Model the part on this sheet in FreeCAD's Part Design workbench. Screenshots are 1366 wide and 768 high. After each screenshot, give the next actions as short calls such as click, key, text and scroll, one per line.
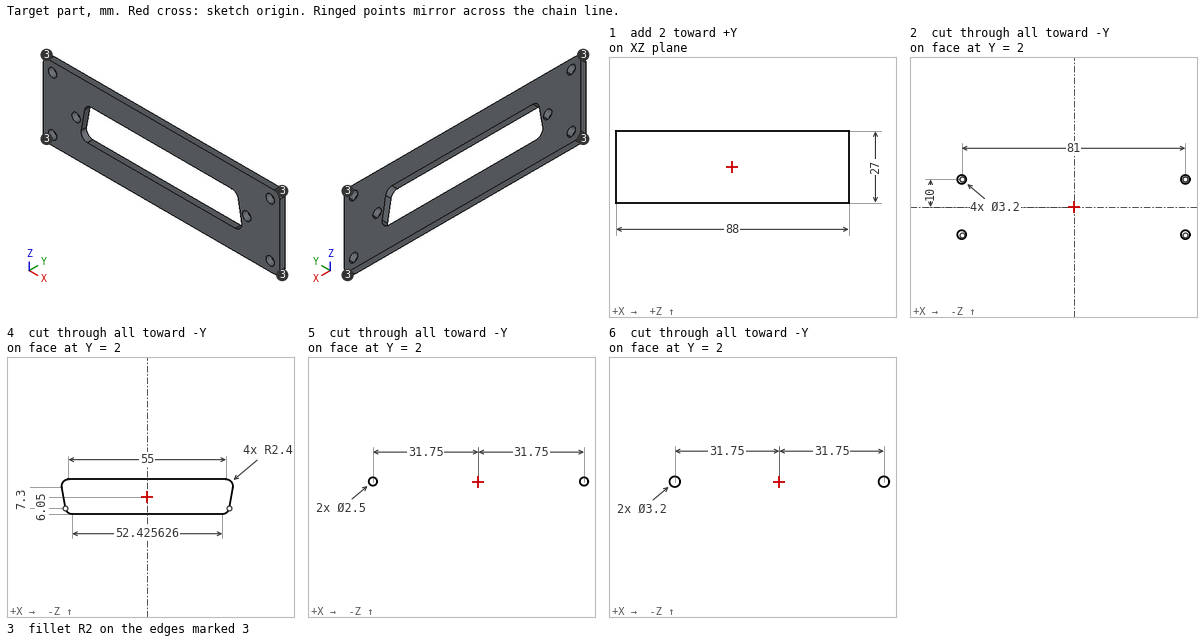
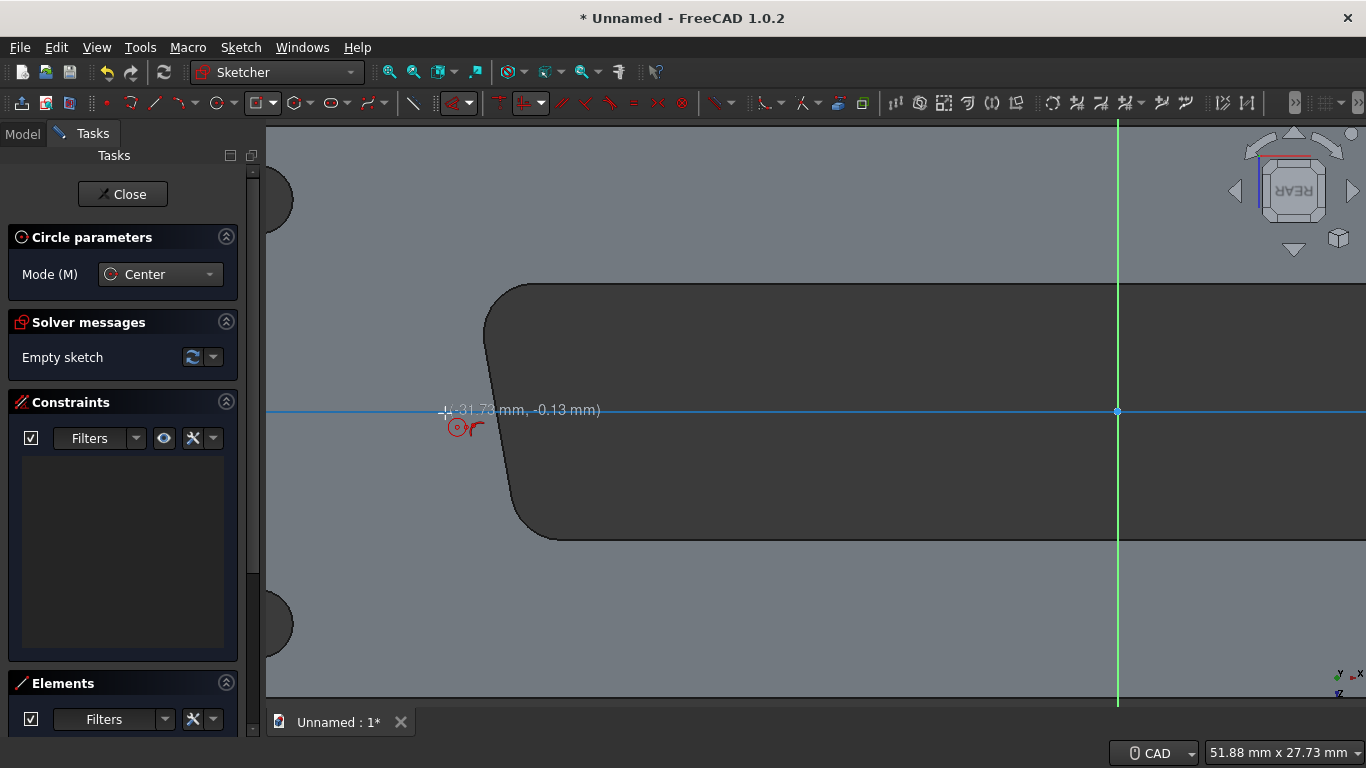
click(444, 412)
click(463, 393)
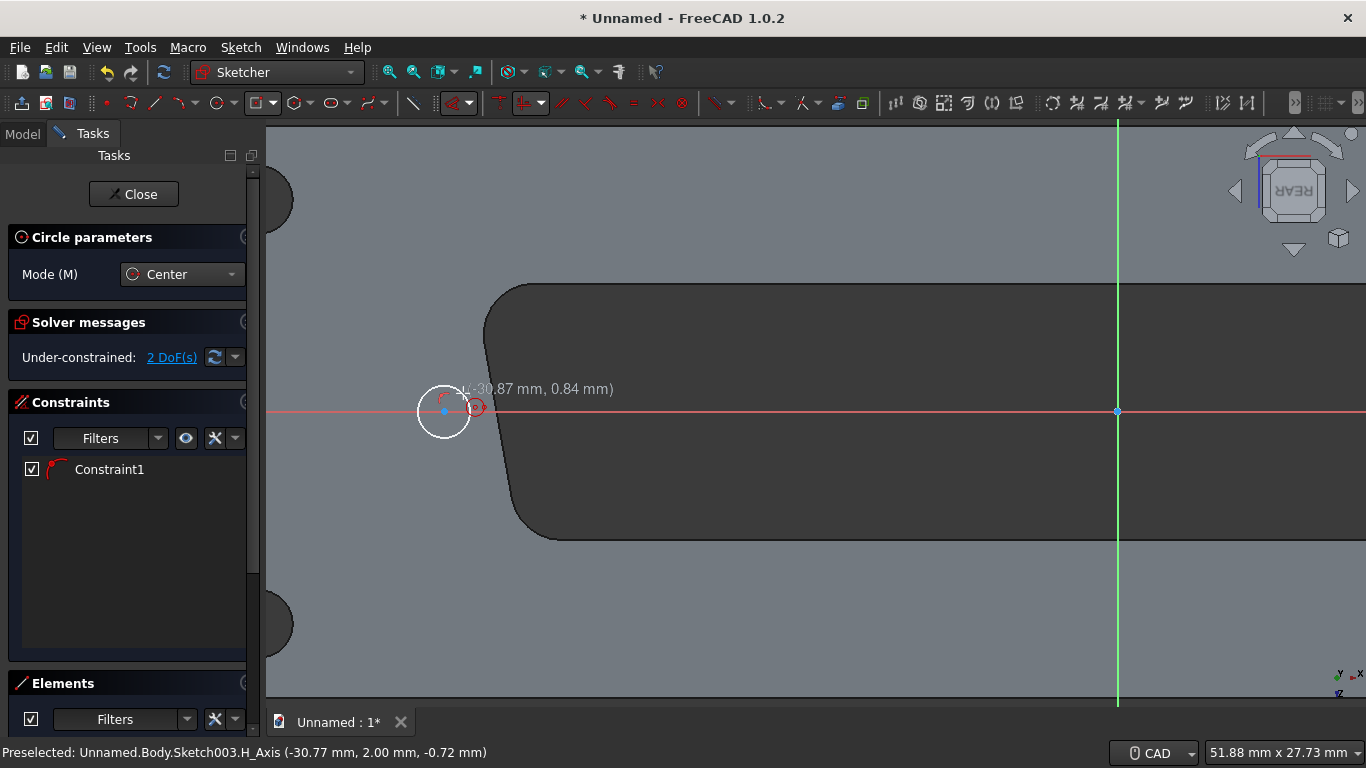
scroll(445, 414, down, 4)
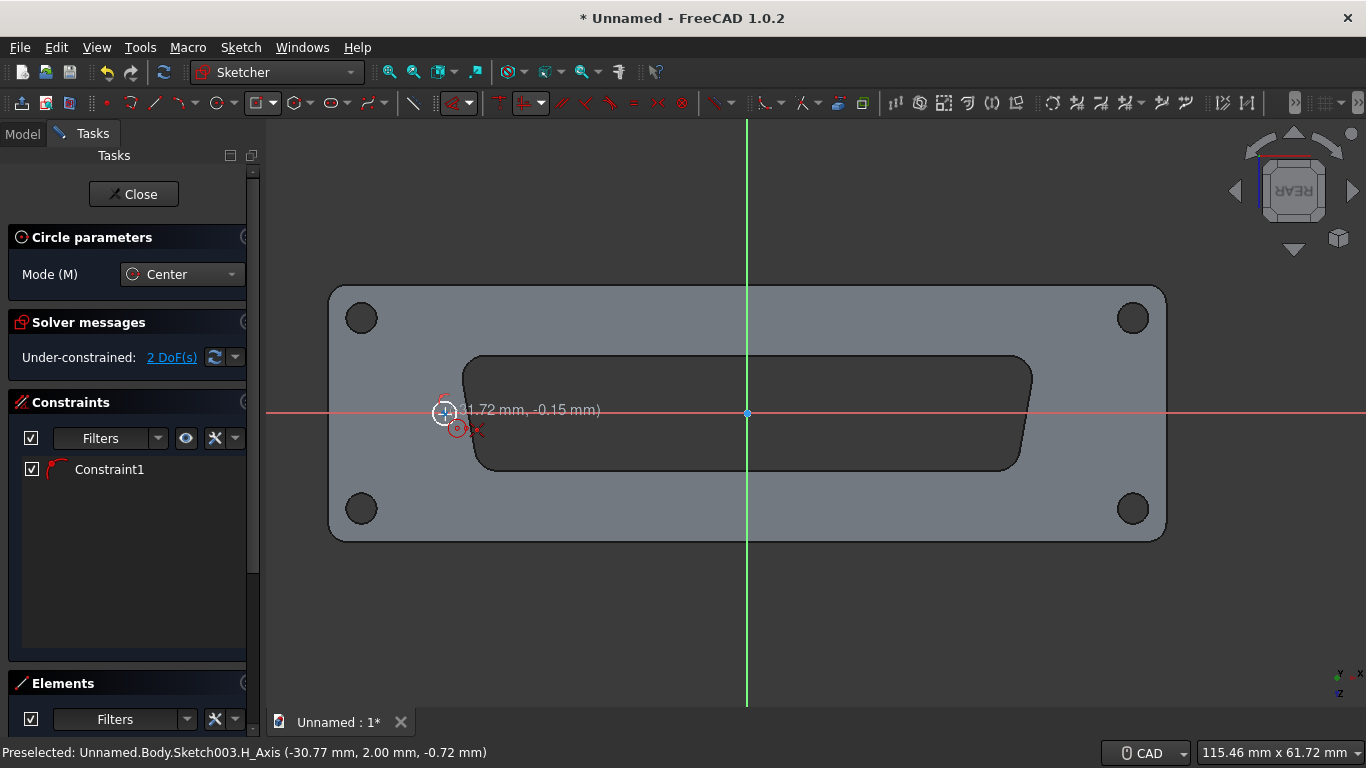
scroll(1050, 413, up, 4)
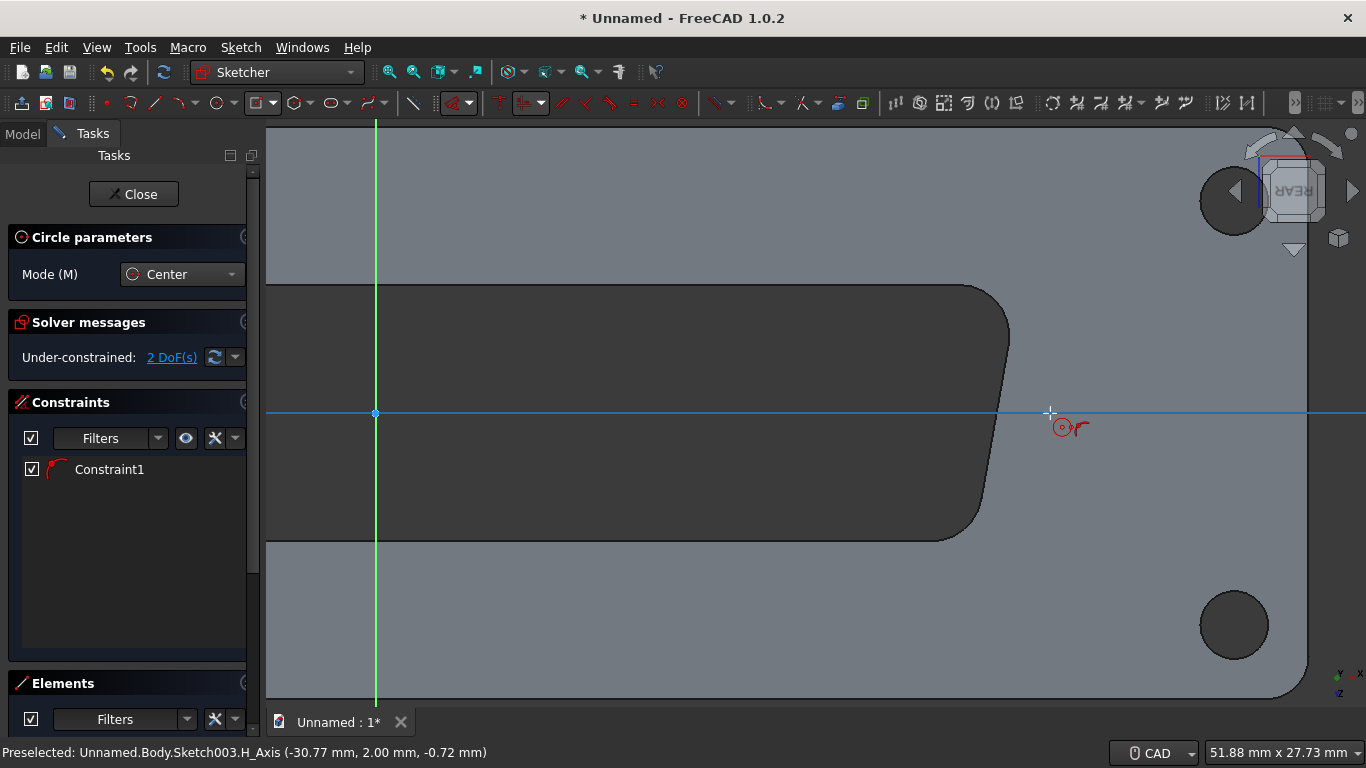
click(1049, 413)
click(1067, 394)
key(Escape)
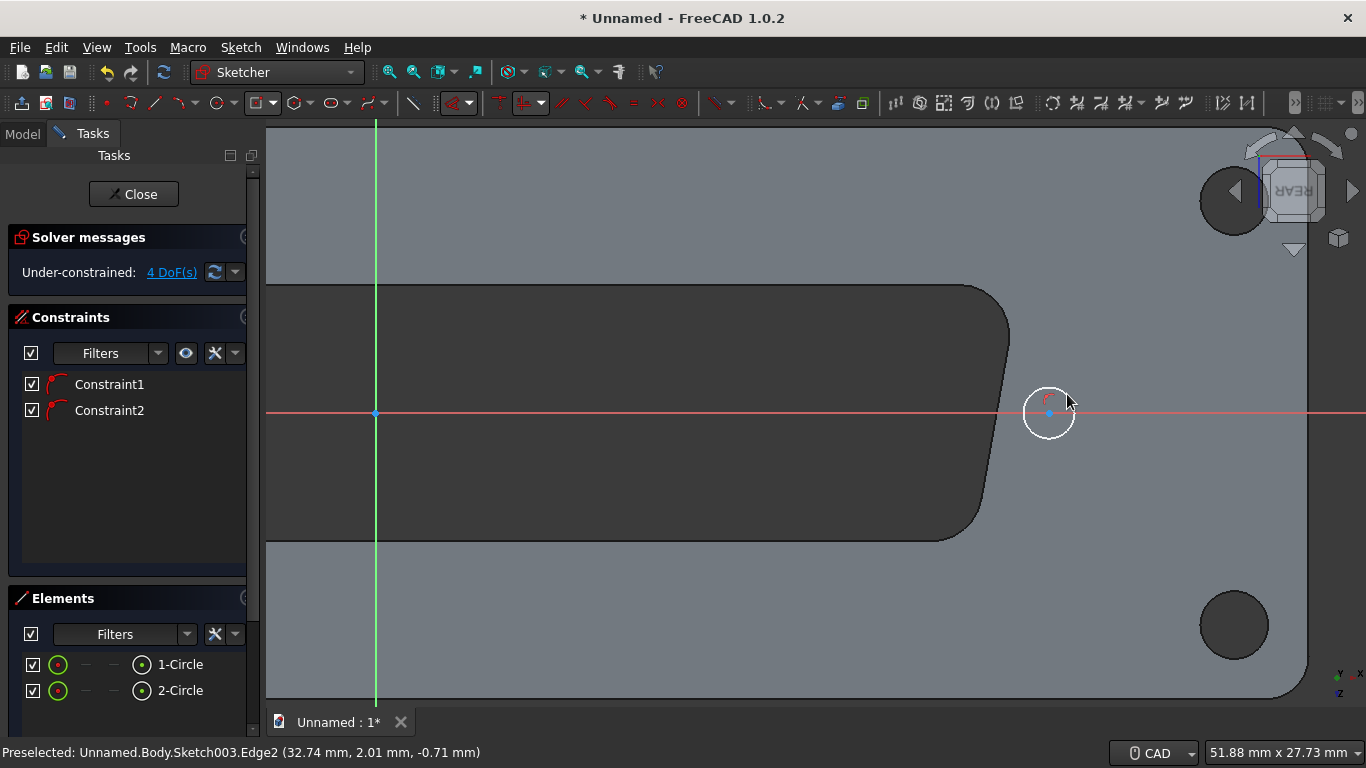
scroll(1051, 413, down, 4)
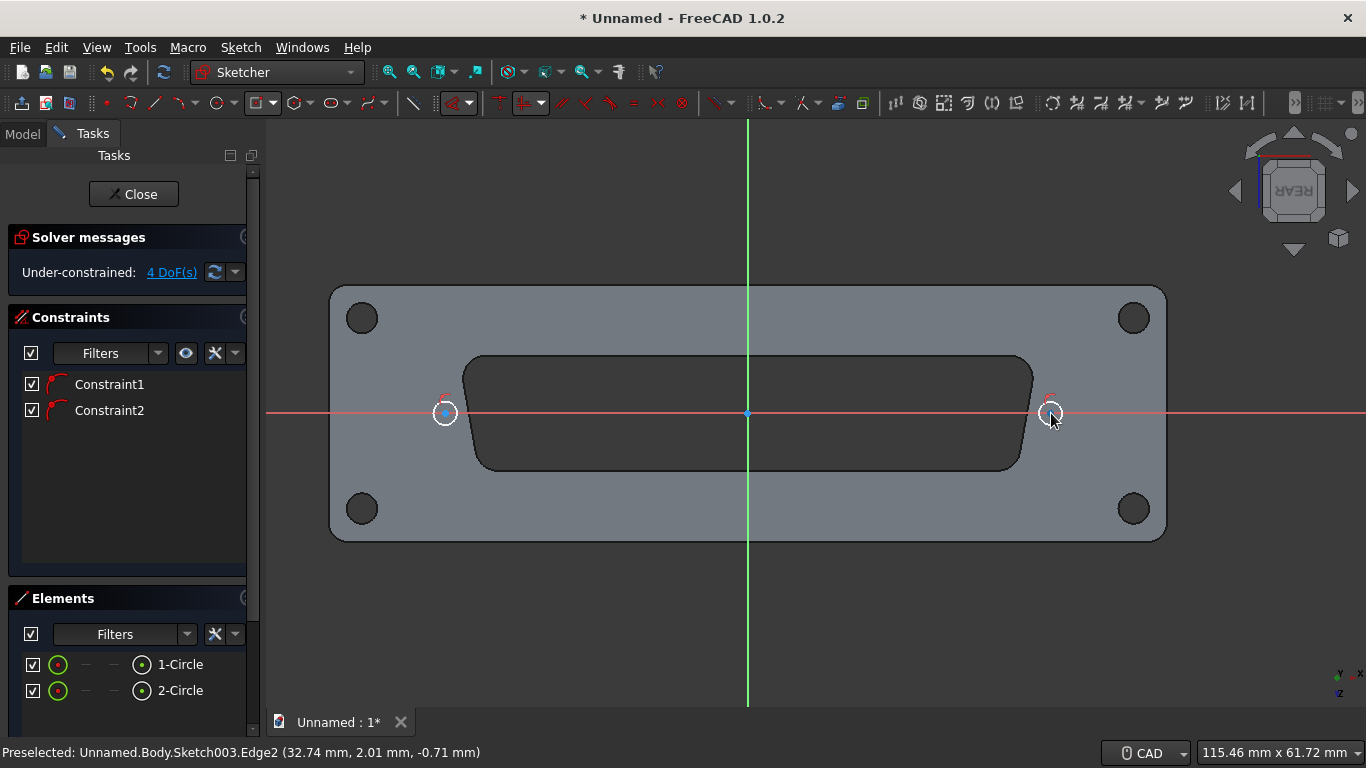
scroll(453, 405, up, 3)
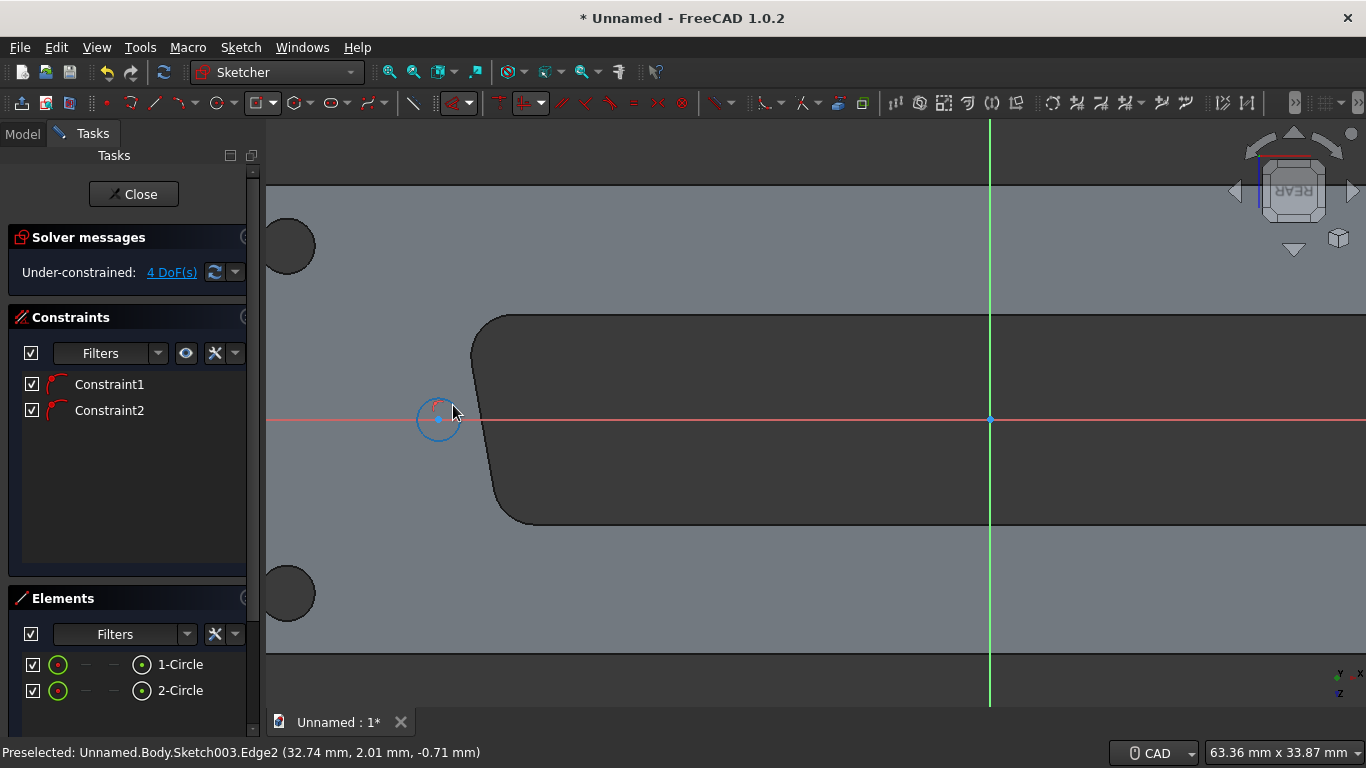
click(454, 405)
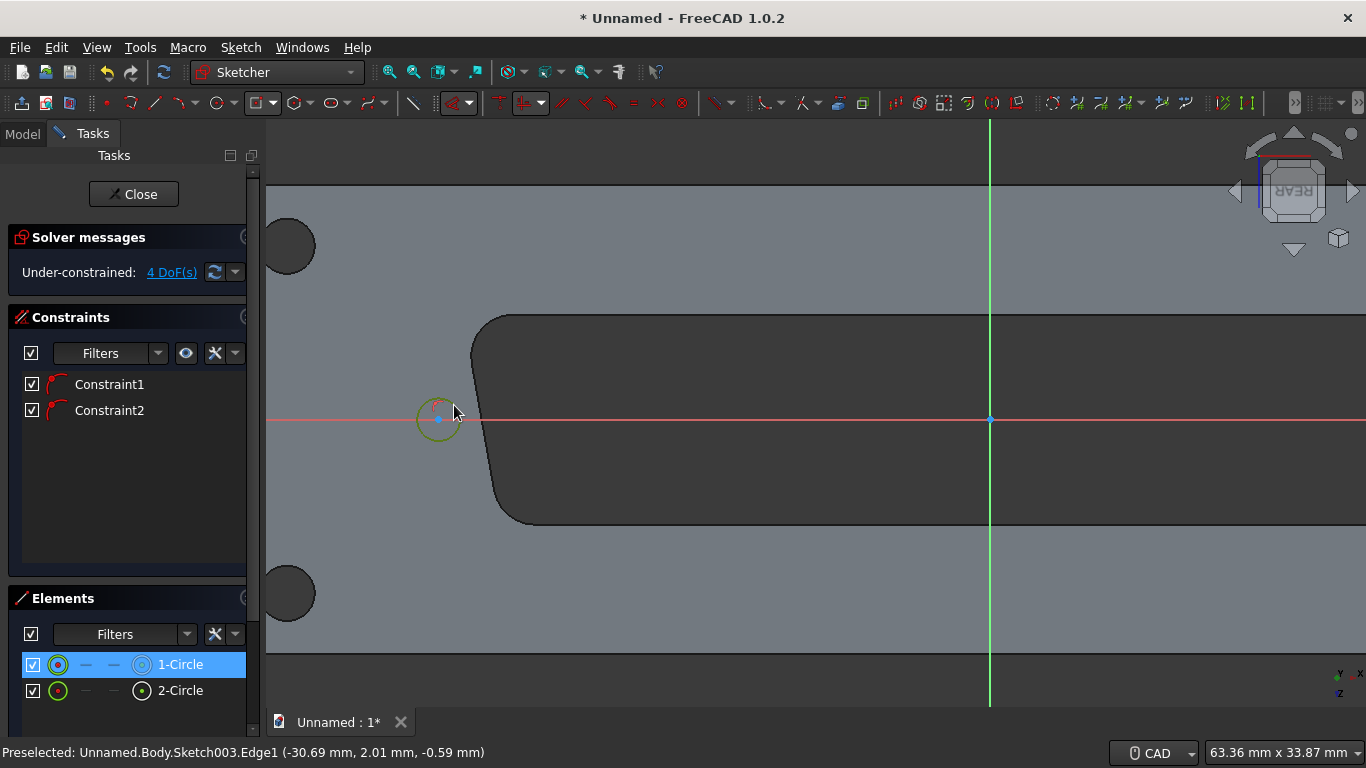
scroll(452, 405, down, 3)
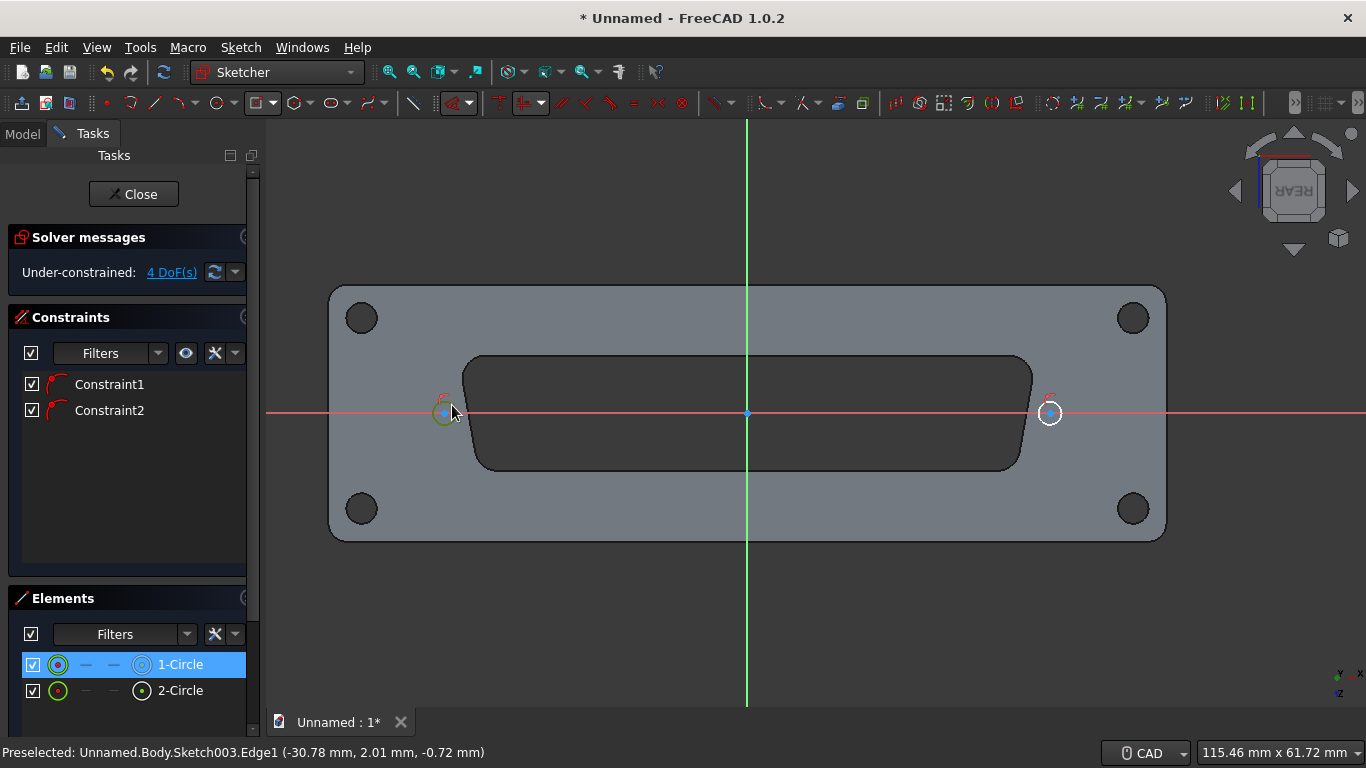
scroll(1058, 405, up, 3)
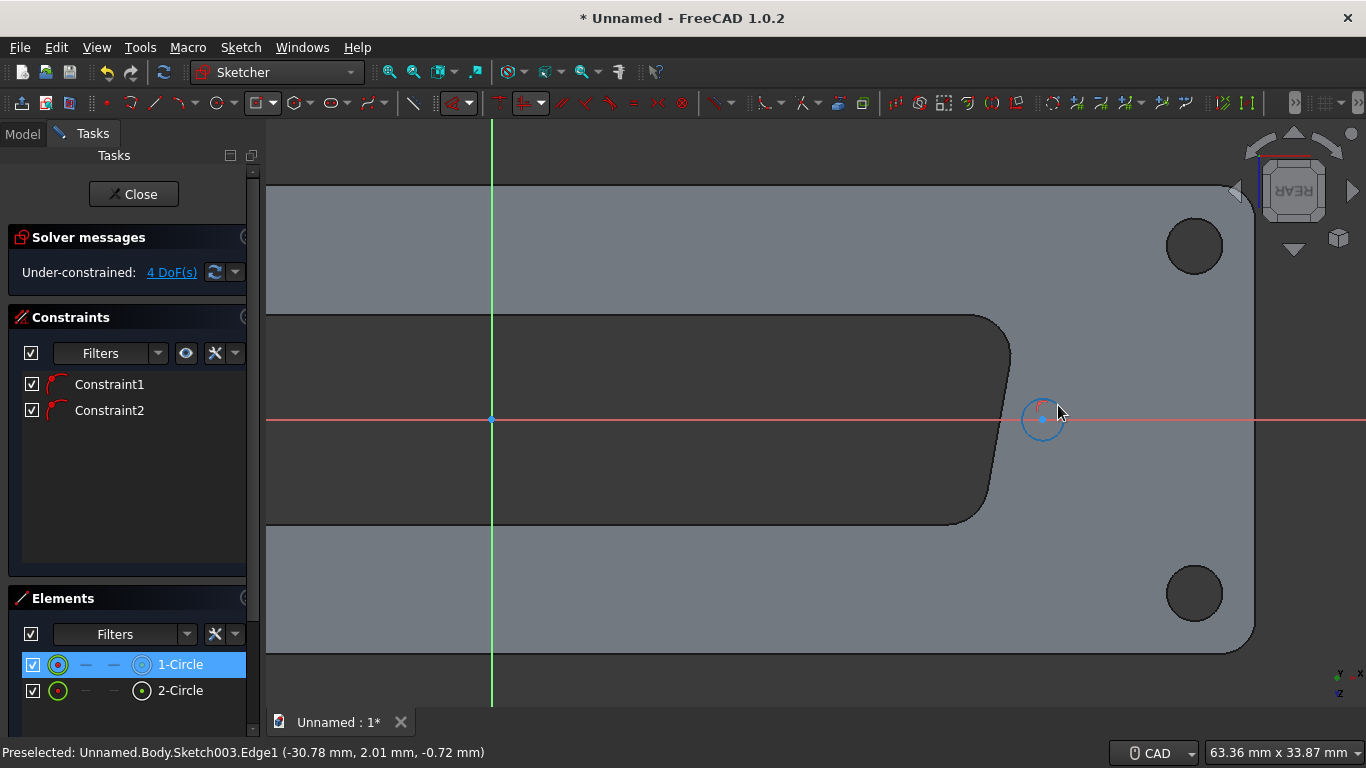
click(1058, 405)